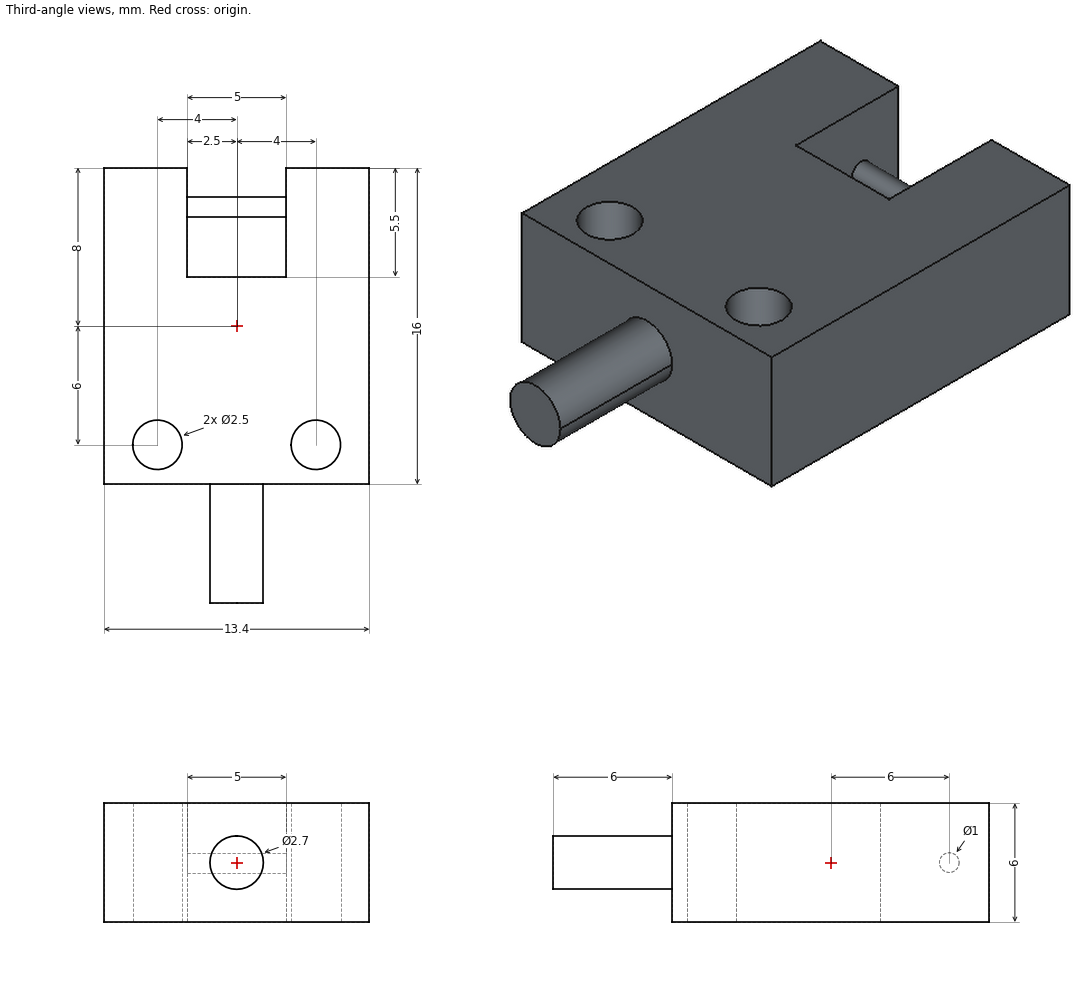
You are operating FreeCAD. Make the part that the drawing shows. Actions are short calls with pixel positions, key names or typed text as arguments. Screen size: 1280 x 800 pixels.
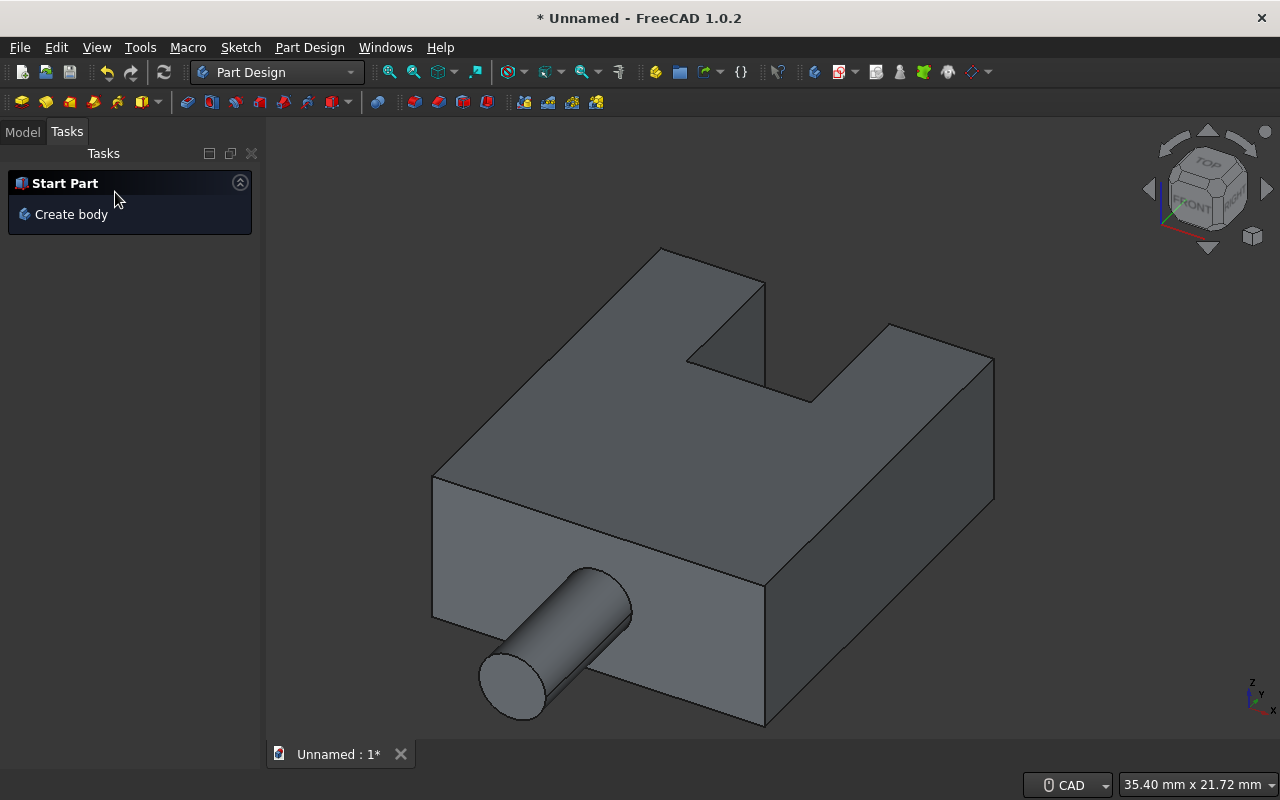
click(390, 72)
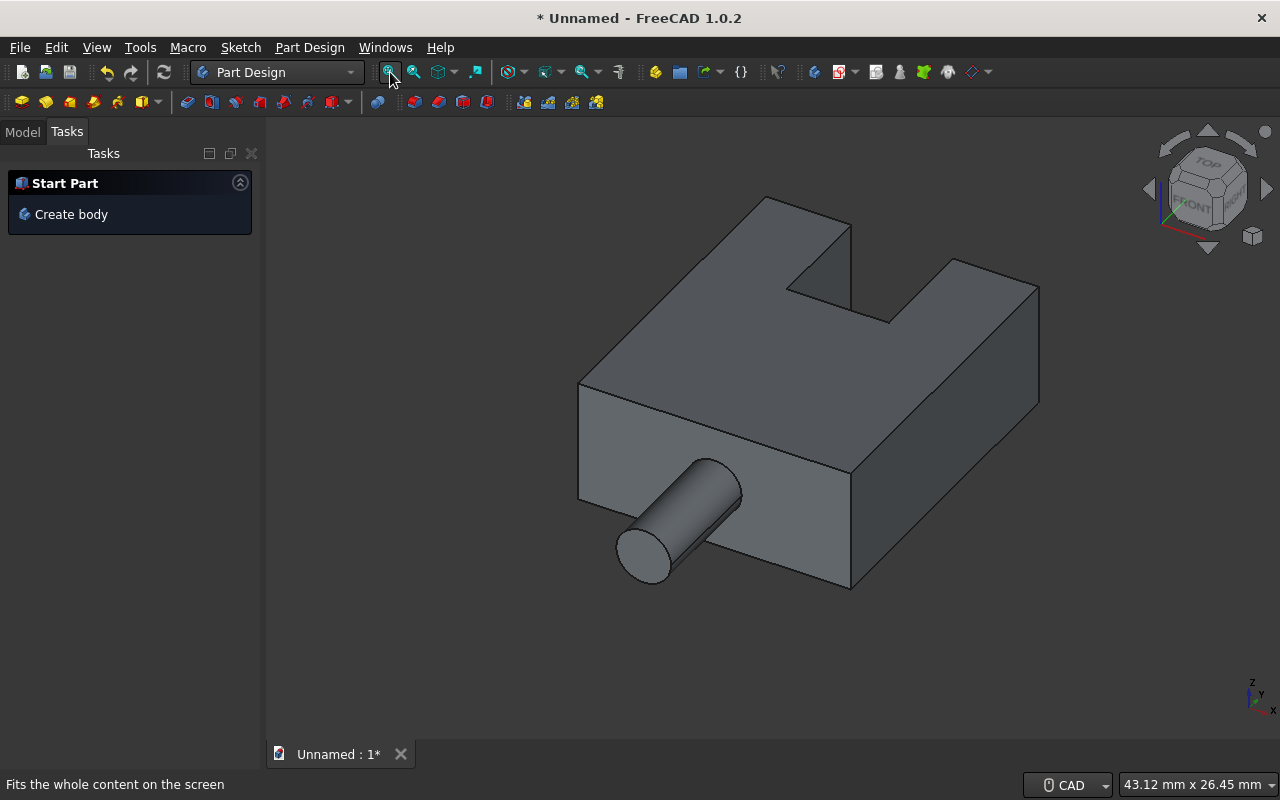
click(820, 374)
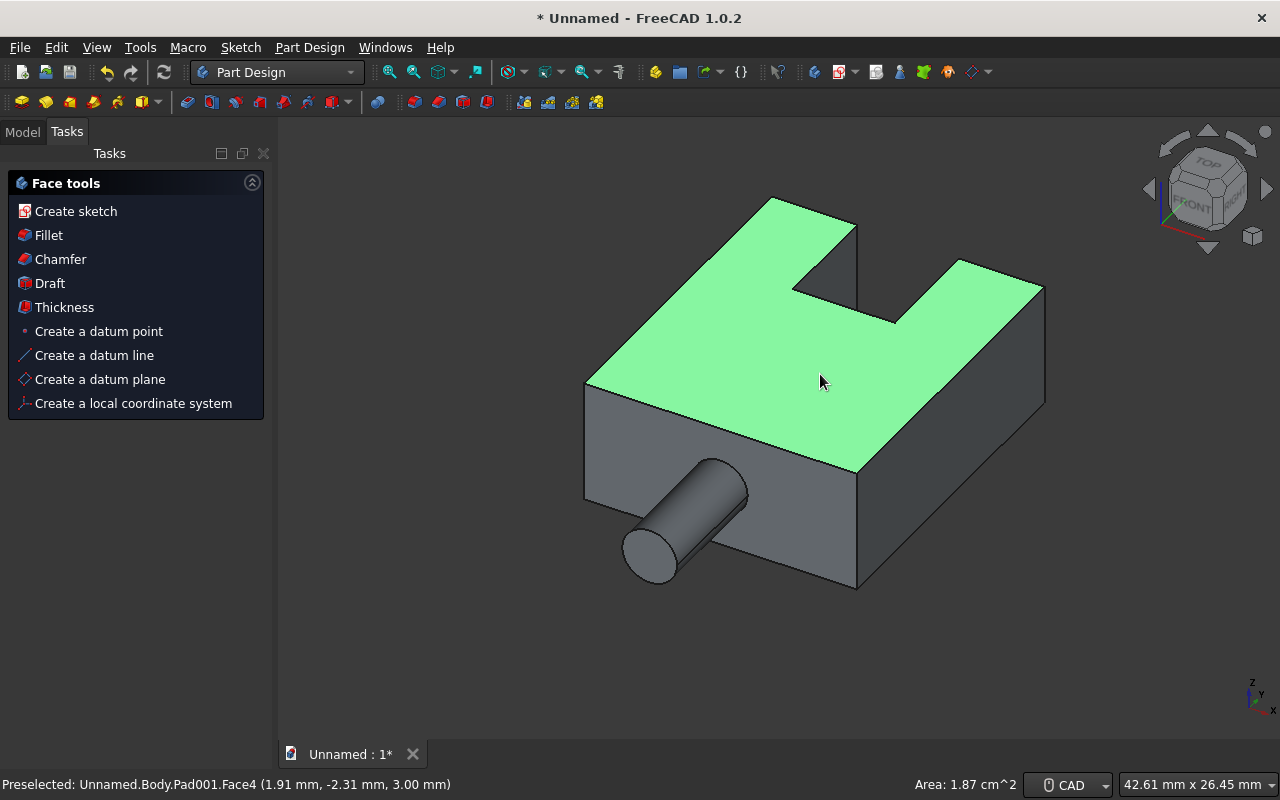
click(840, 72)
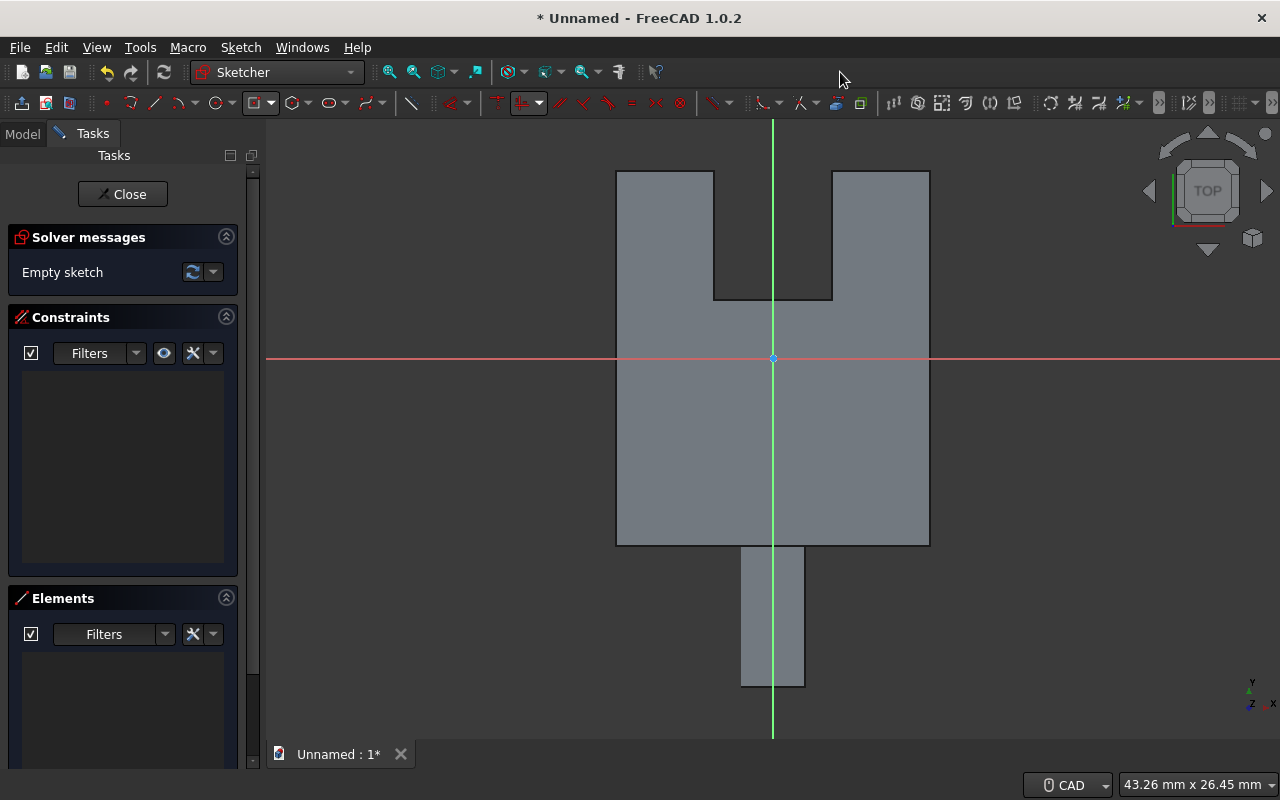
scroll(829, 456, up, 4)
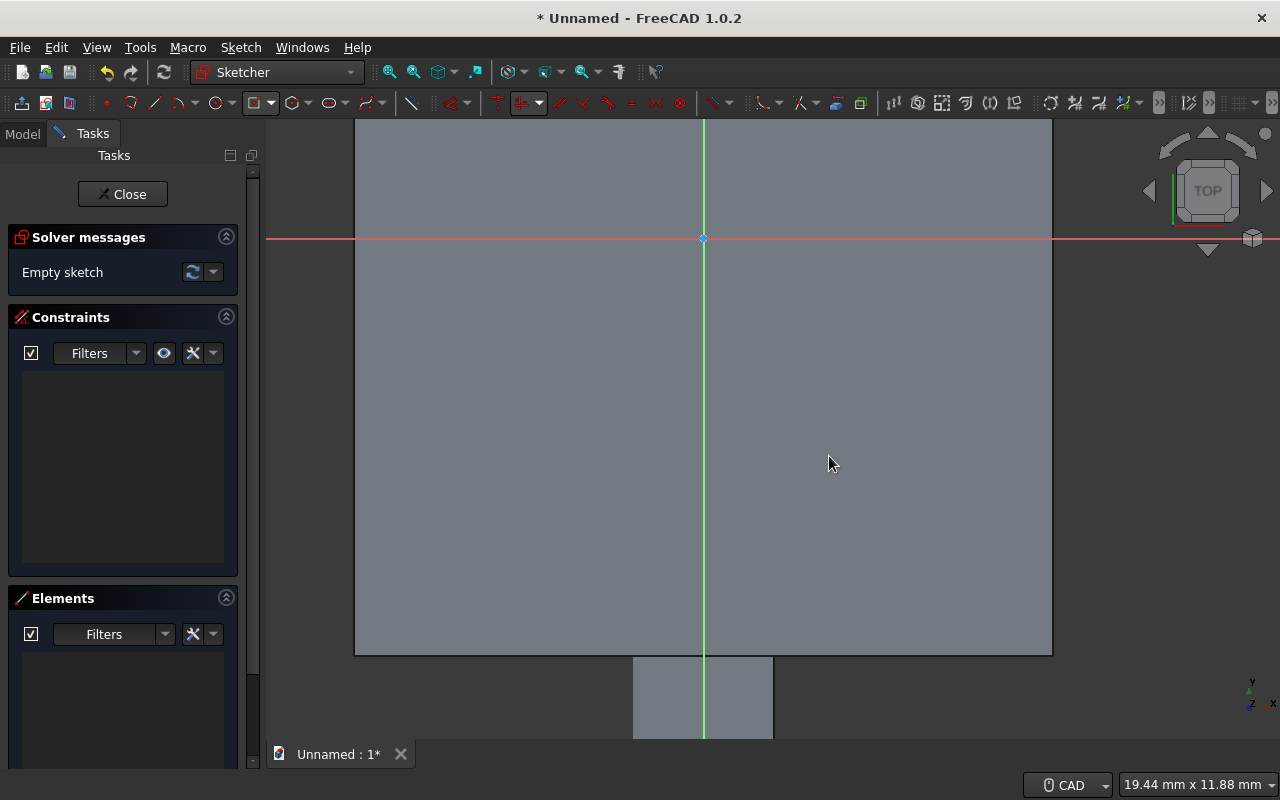
key(g)
key(c)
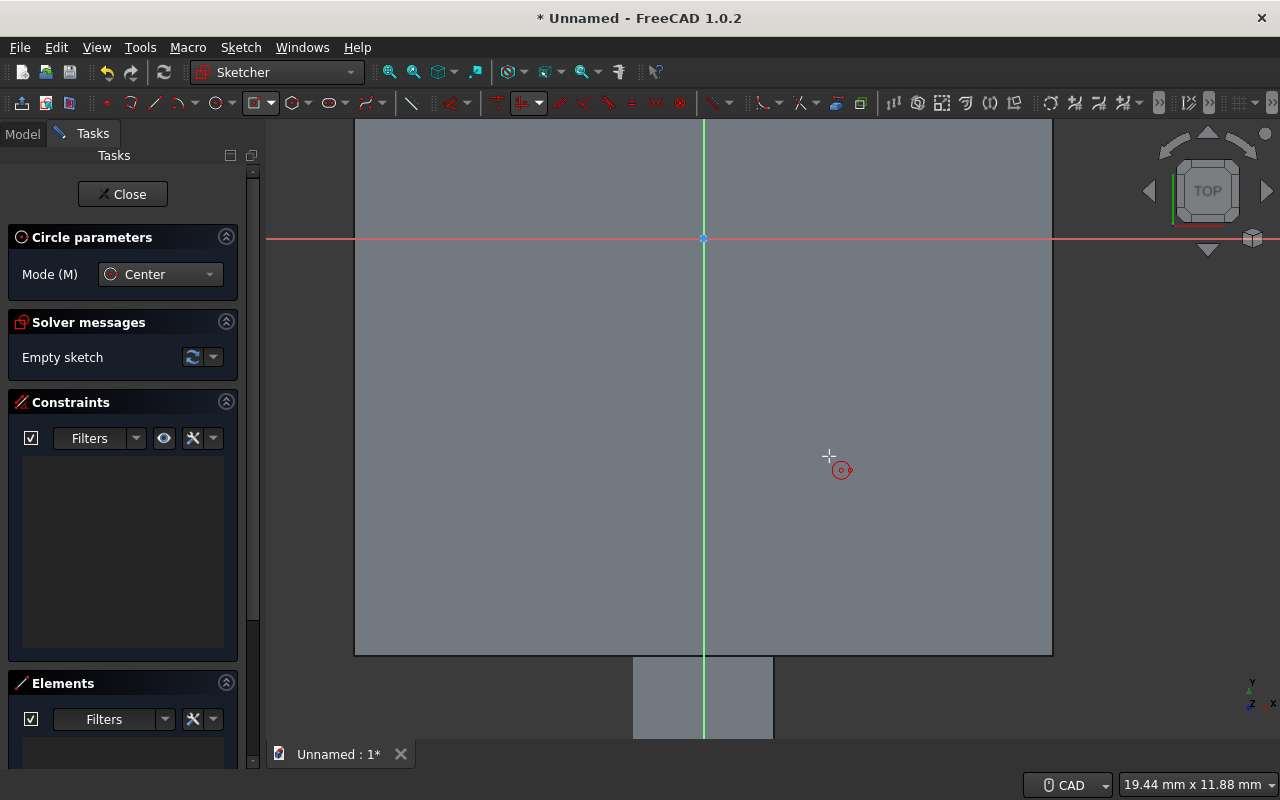
click(495, 552)
move(541, 506)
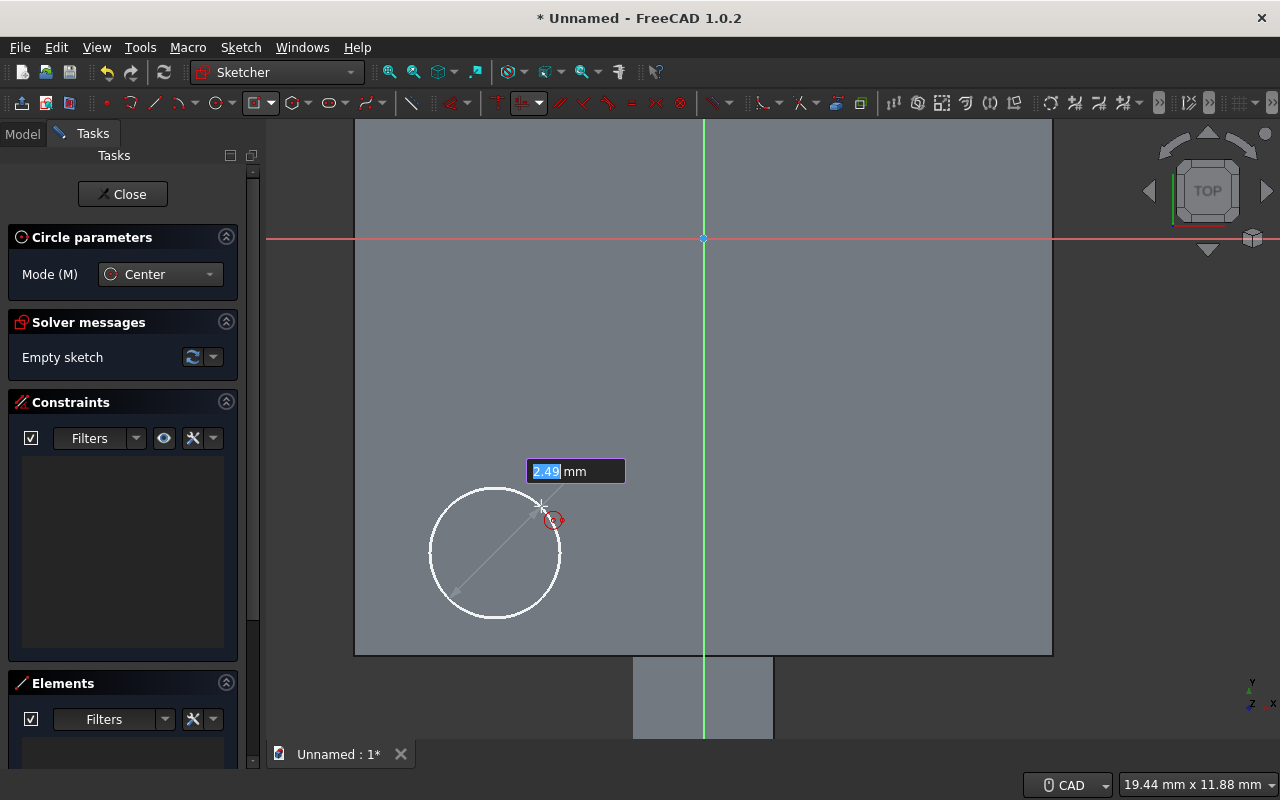
text(2.5)
key(Return)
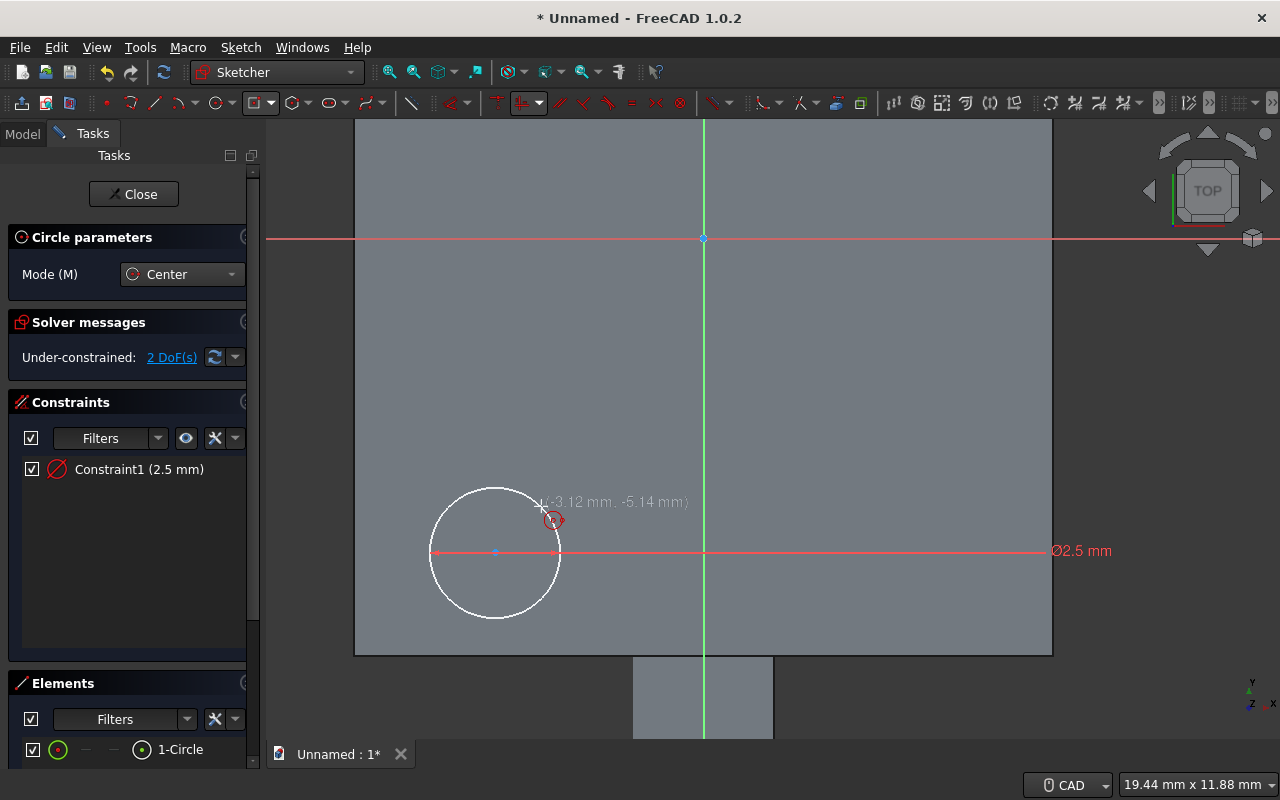
click(912, 552)
move(958, 506)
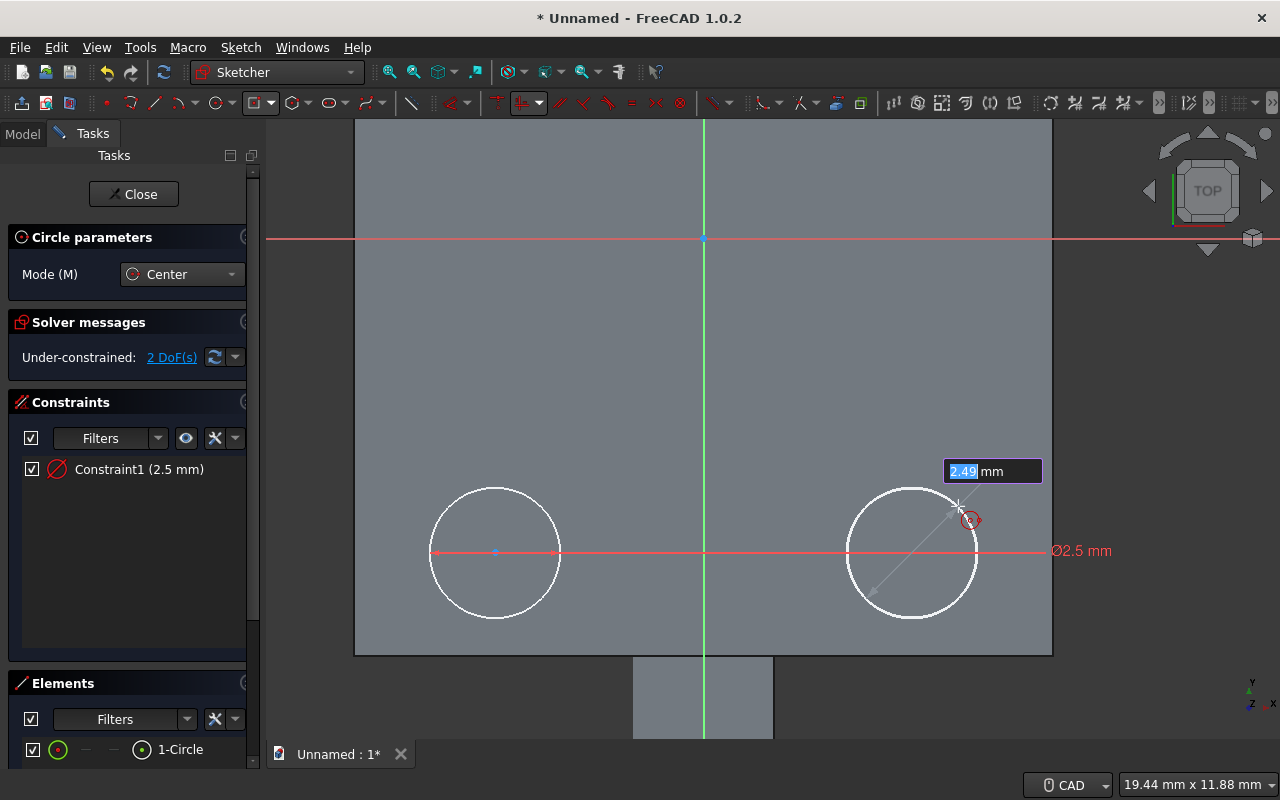
text(2.5)
key(Return)
key(Escape)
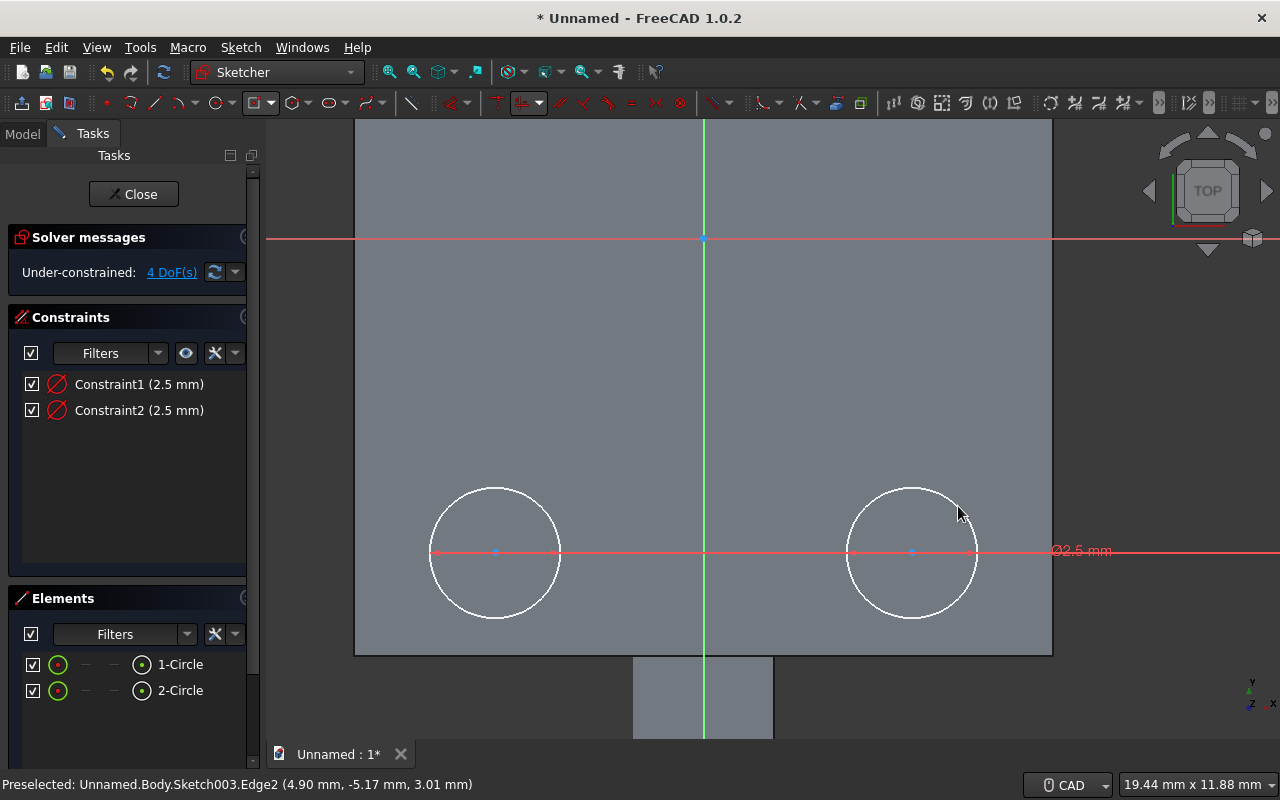
click(495, 553)